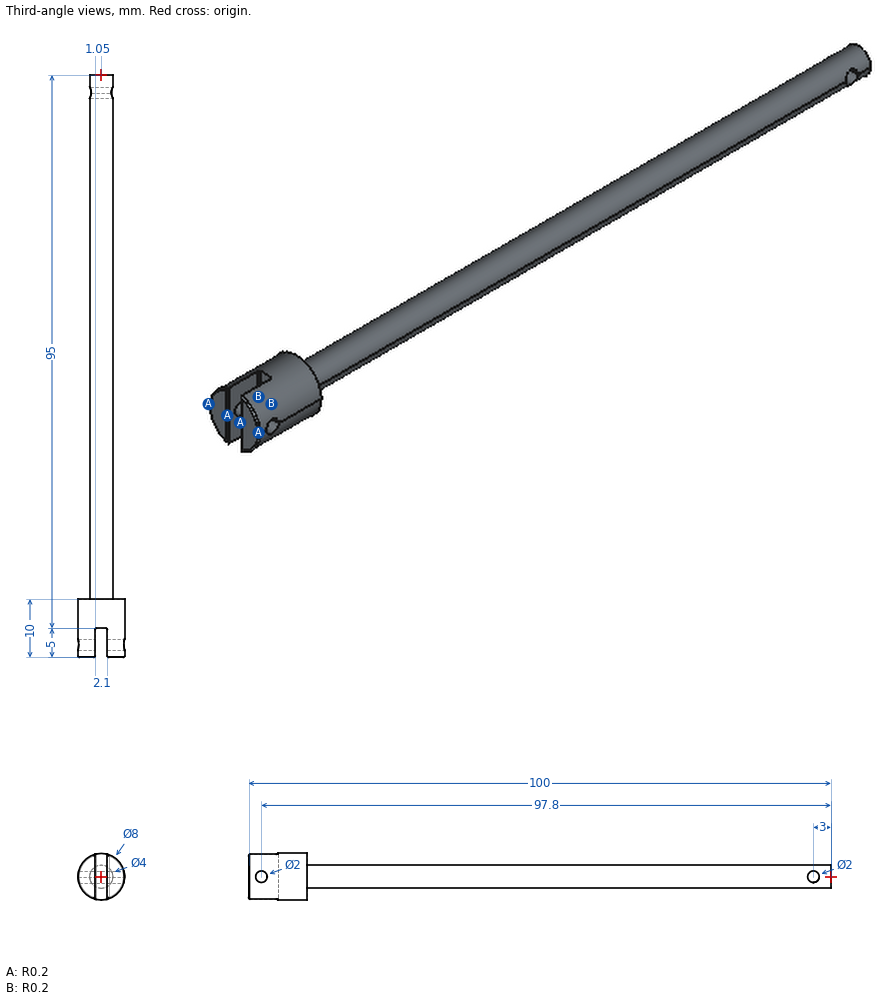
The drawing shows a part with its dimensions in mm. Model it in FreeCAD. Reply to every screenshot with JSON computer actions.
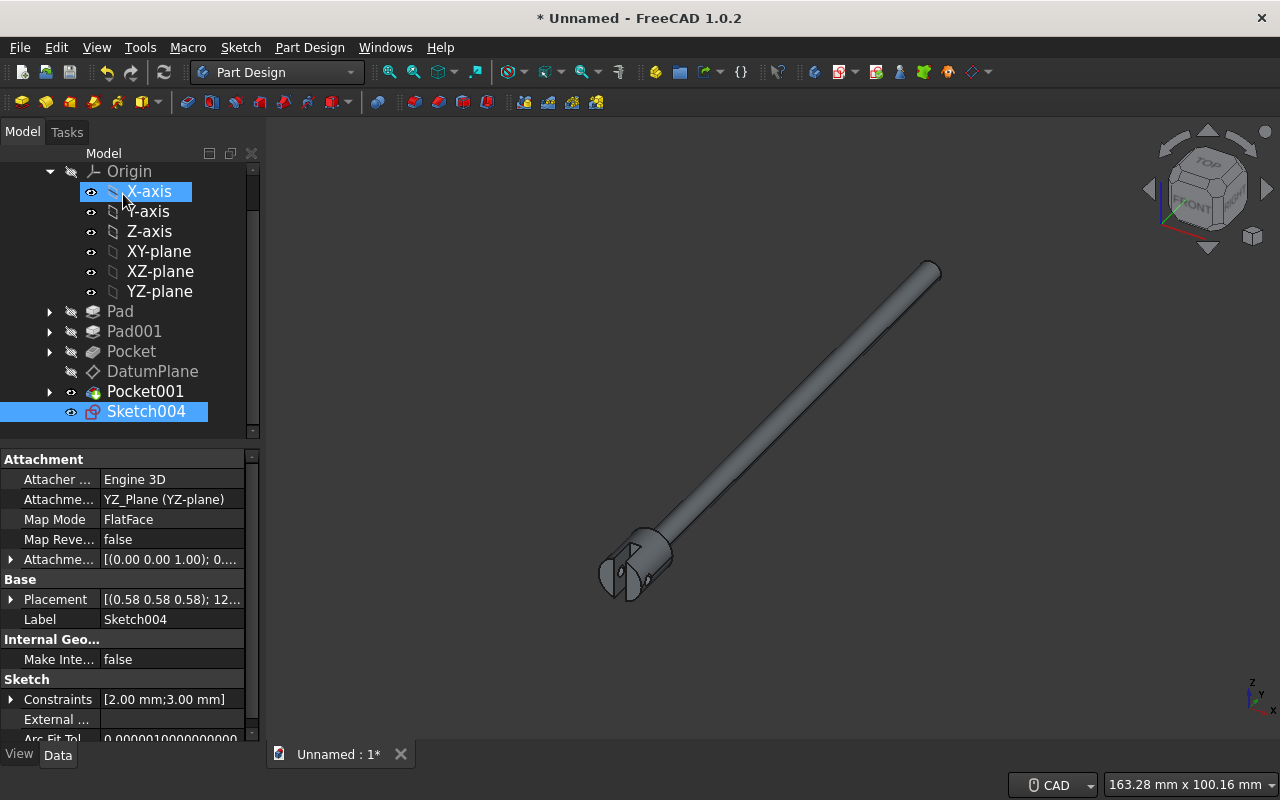
{"action": "left_click", "coordinate": [188, 102]}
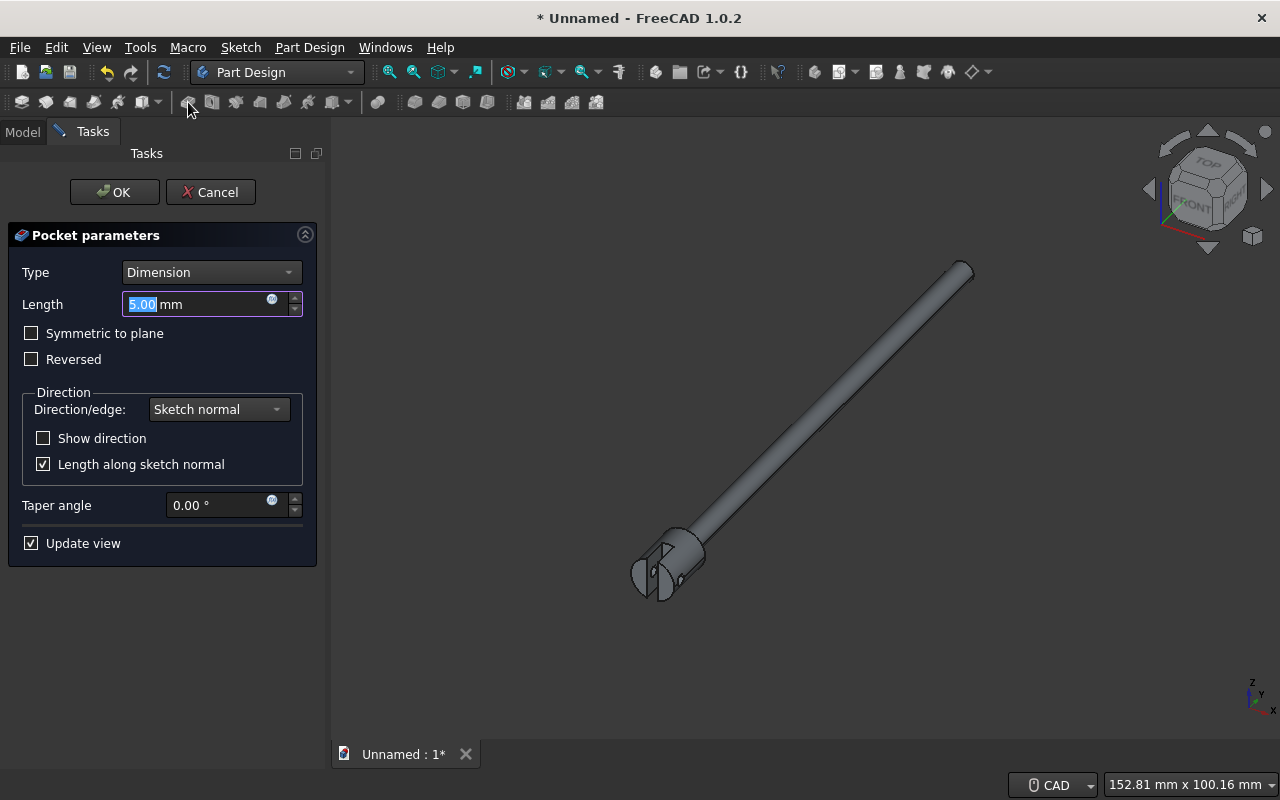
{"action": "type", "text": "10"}
{"action": "key", "text": "Tab"}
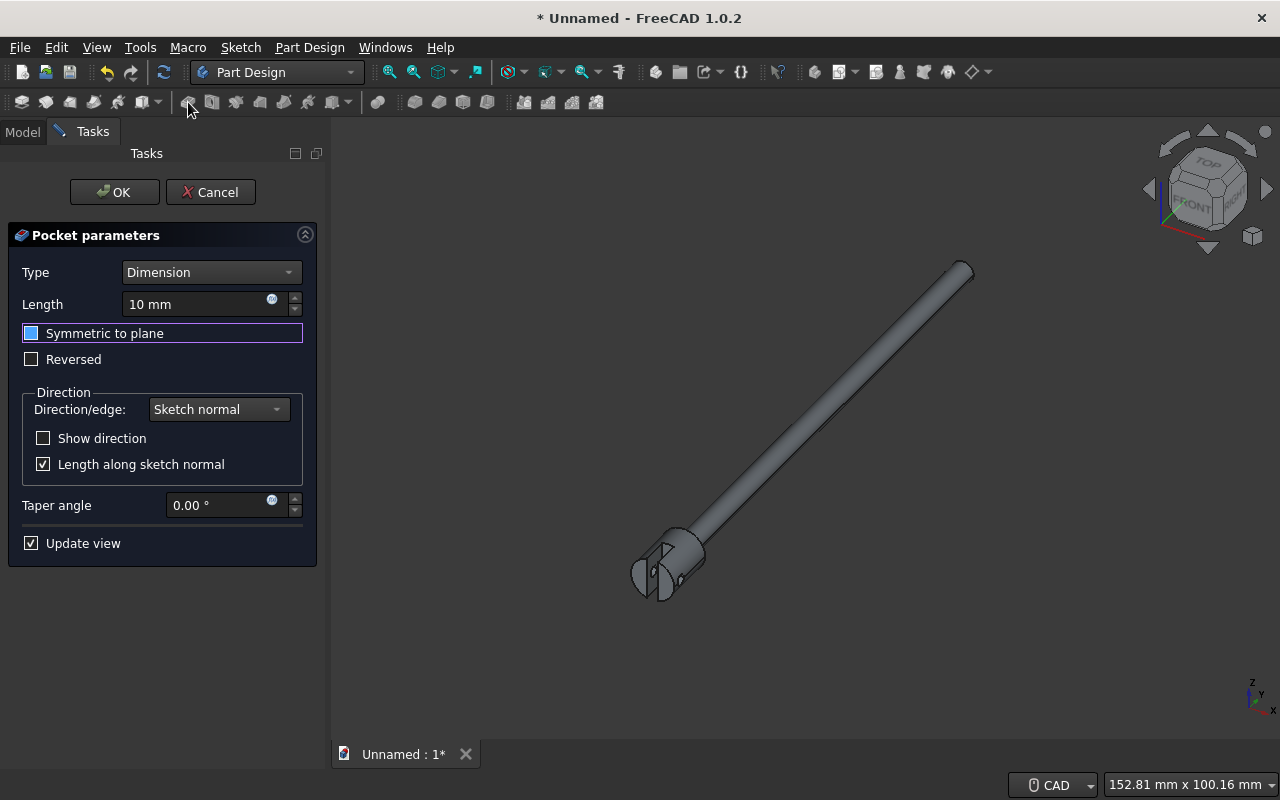
{"action": "left_click", "coordinate": [30, 333]}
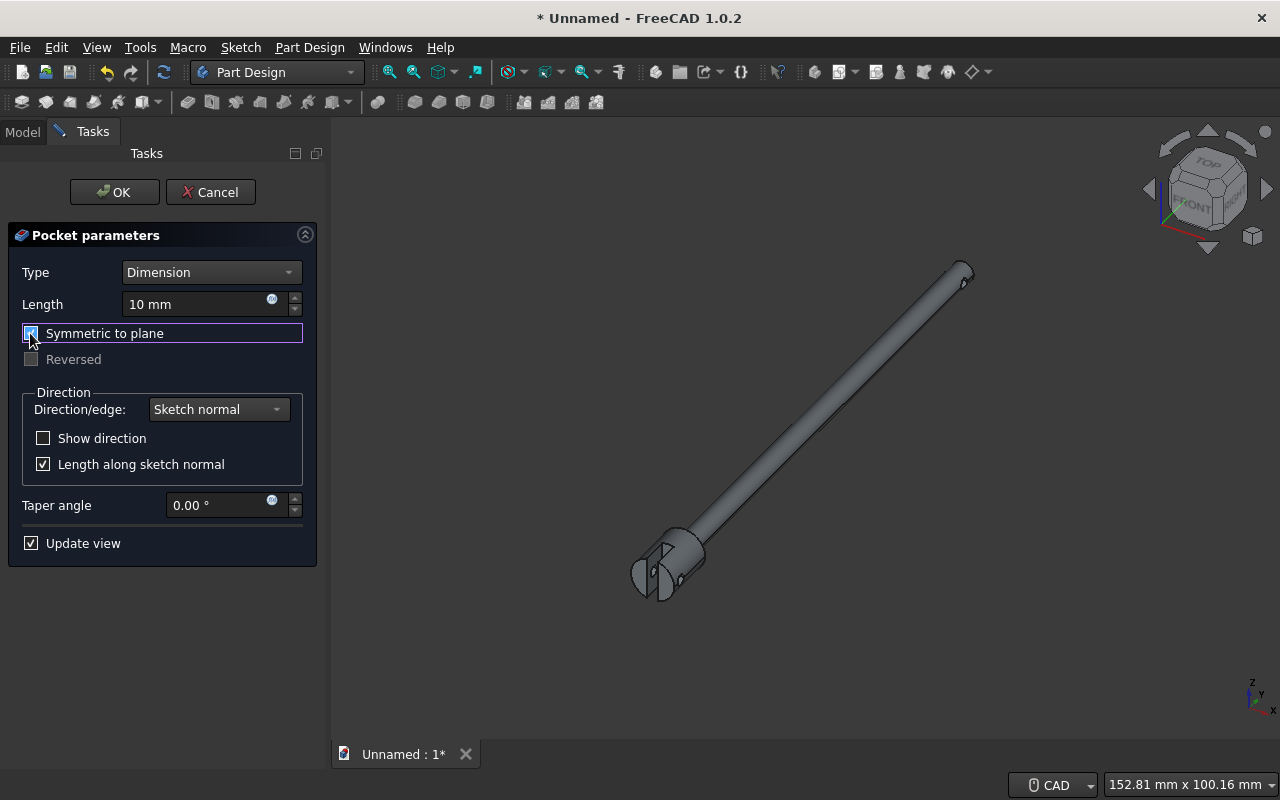
{"action": "left_click", "coordinate": [115, 192]}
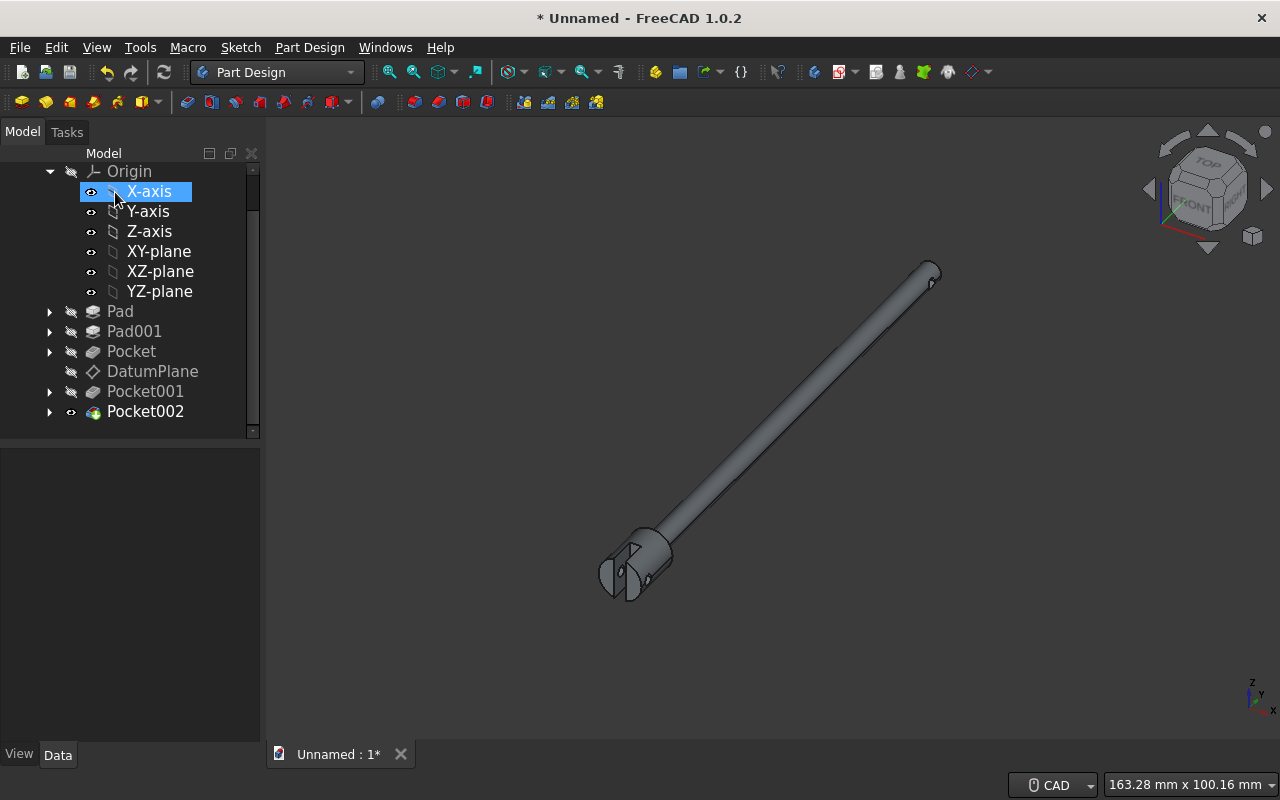
{"action": "left_click", "coordinate": [599, 572]}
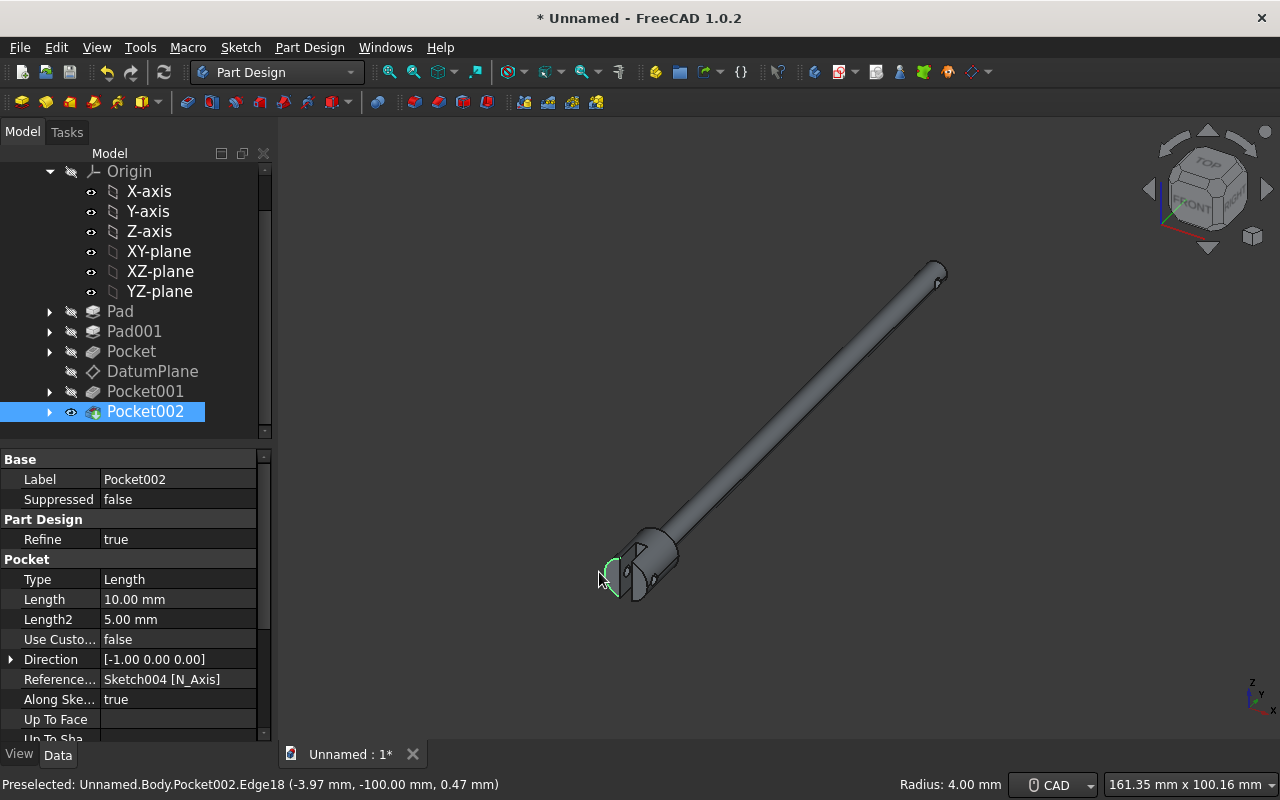
{"action": "left_click", "coordinate": [620, 577], "text": "ctrl"}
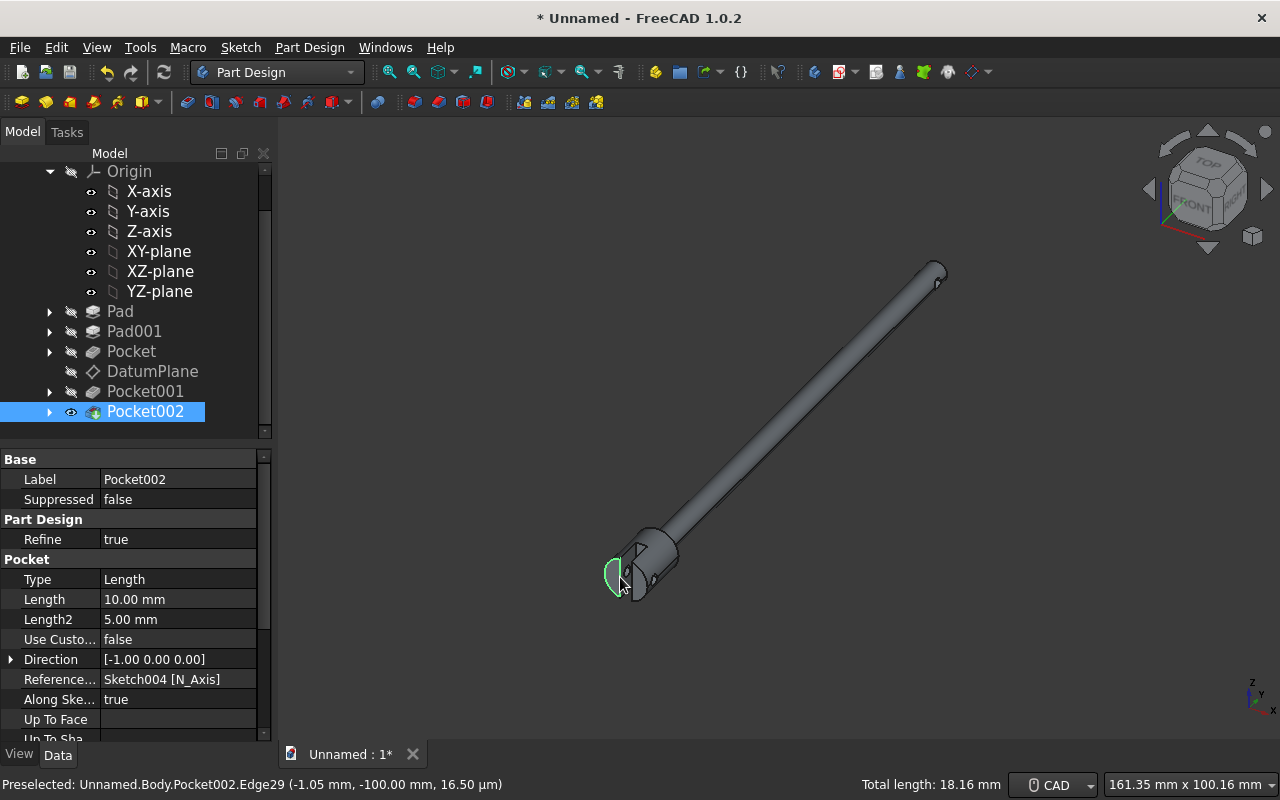
{"action": "left_click", "coordinate": [643, 572], "text": "ctrl"}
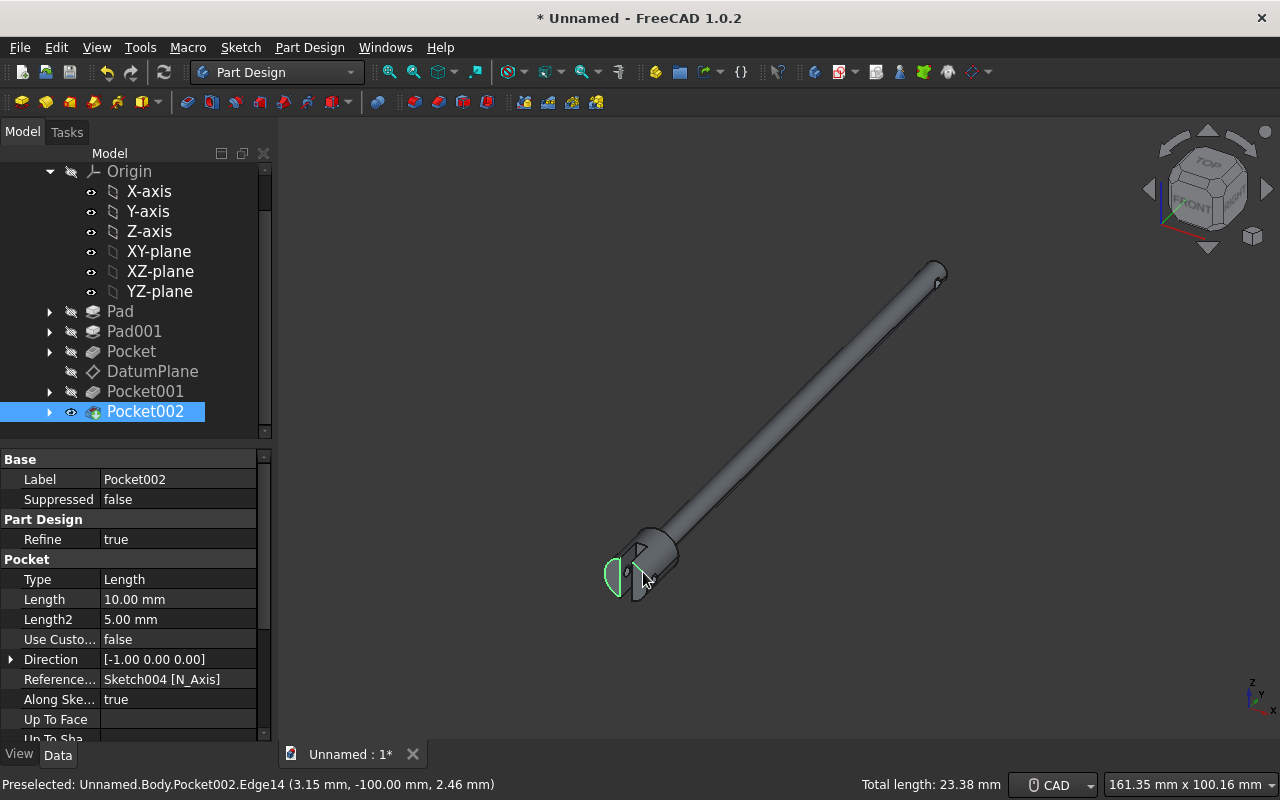
{"action": "key", "text": "0"}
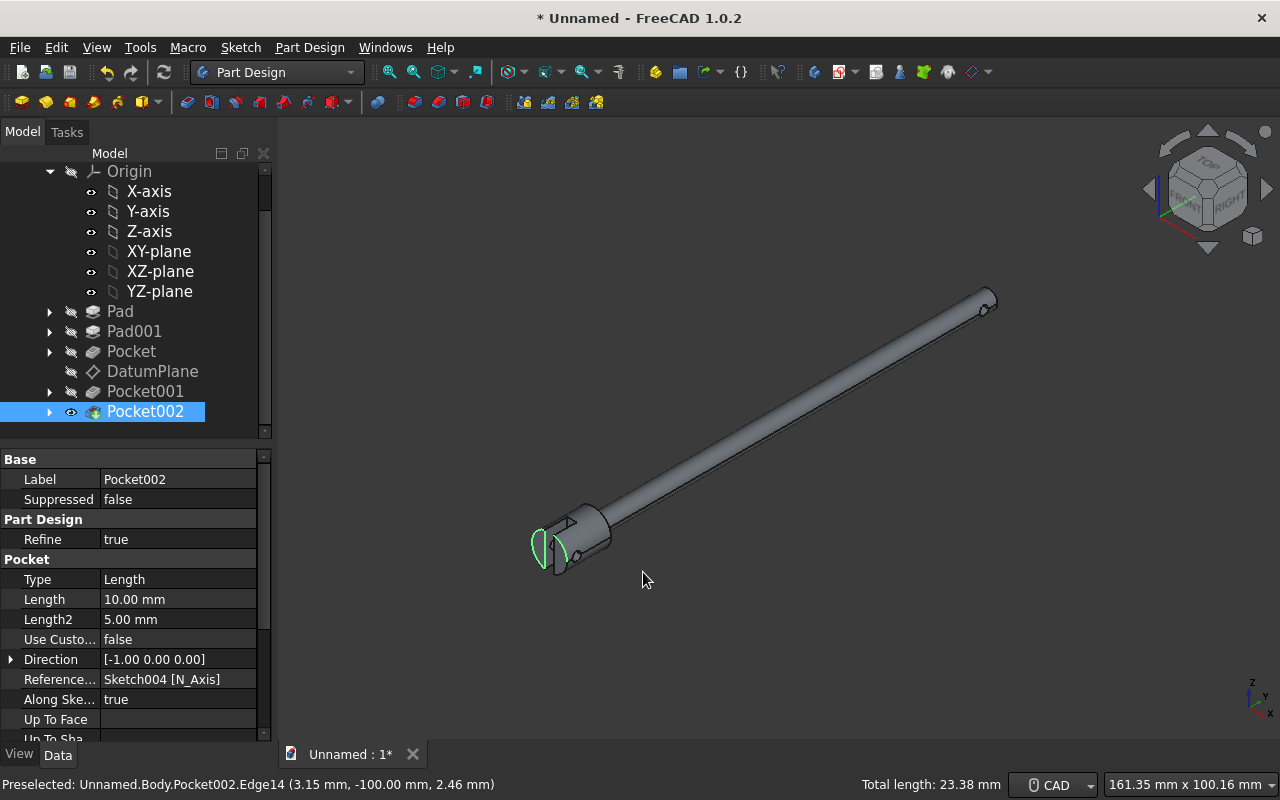
{"action": "key", "text": "2"}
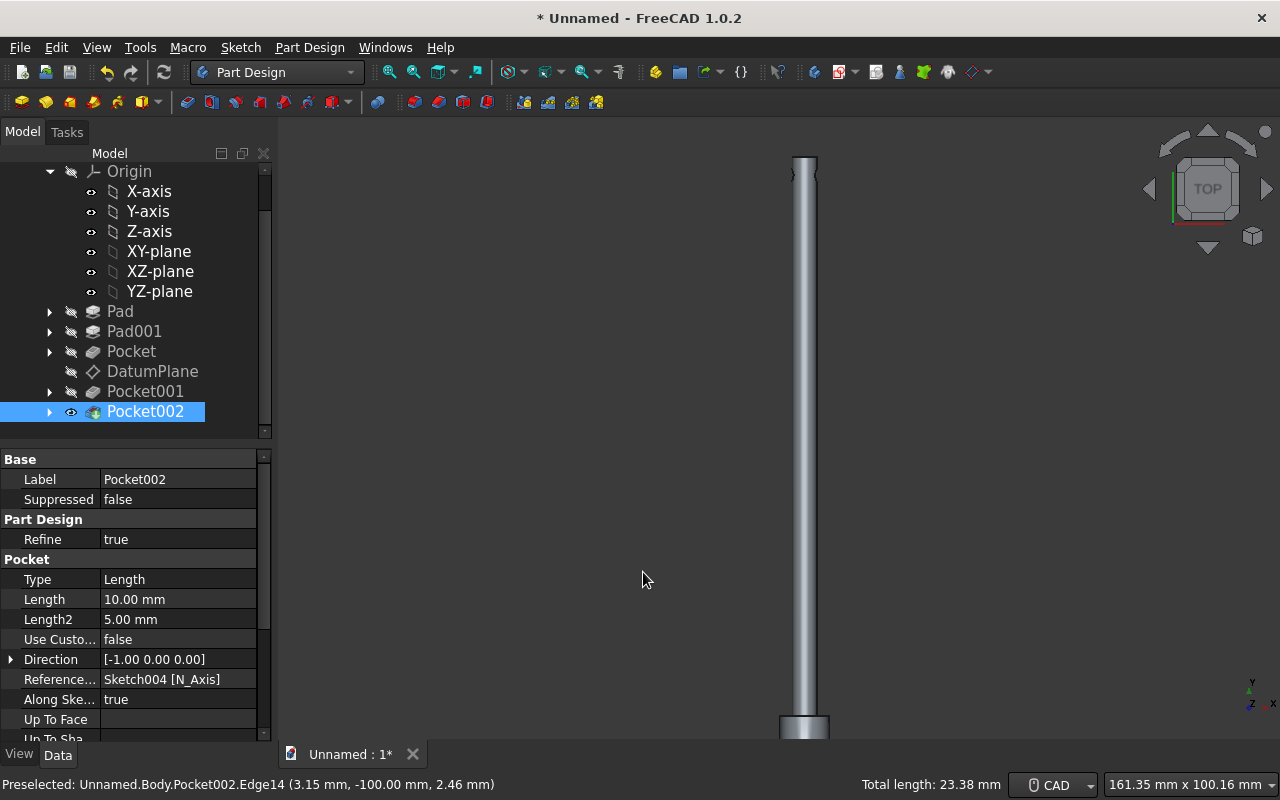
{"action": "key", "text": "v f"}